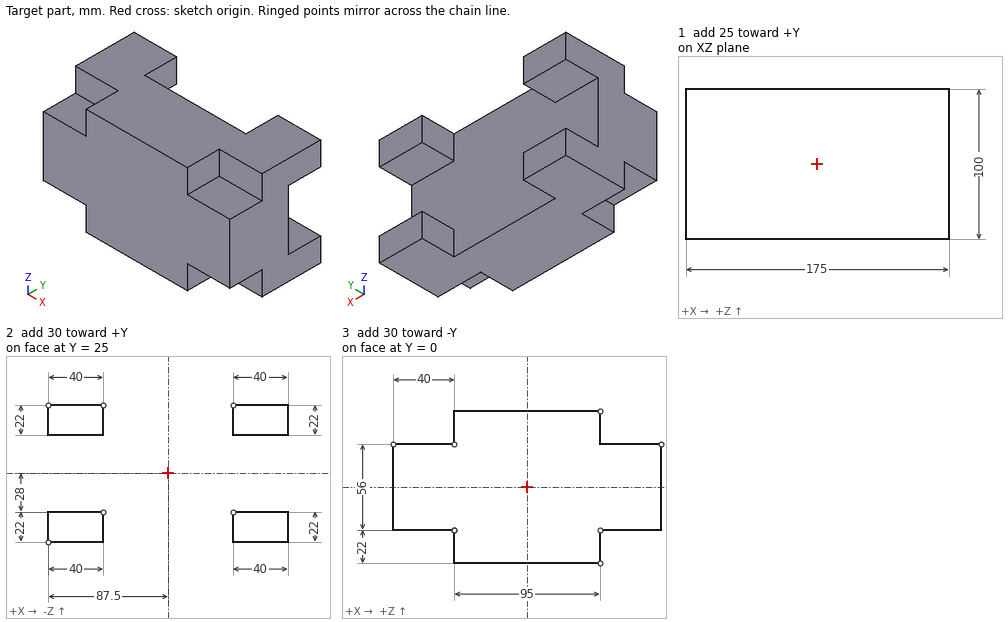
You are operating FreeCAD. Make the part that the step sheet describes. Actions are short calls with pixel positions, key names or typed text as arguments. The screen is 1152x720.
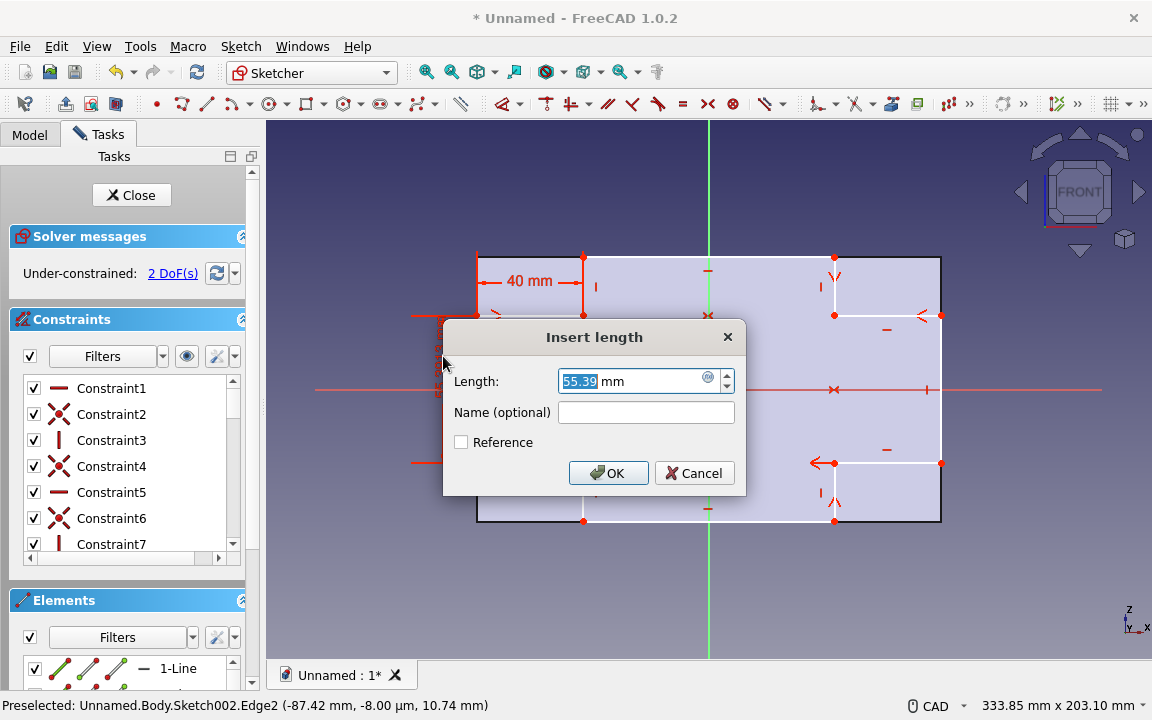
text(56)
key(Return)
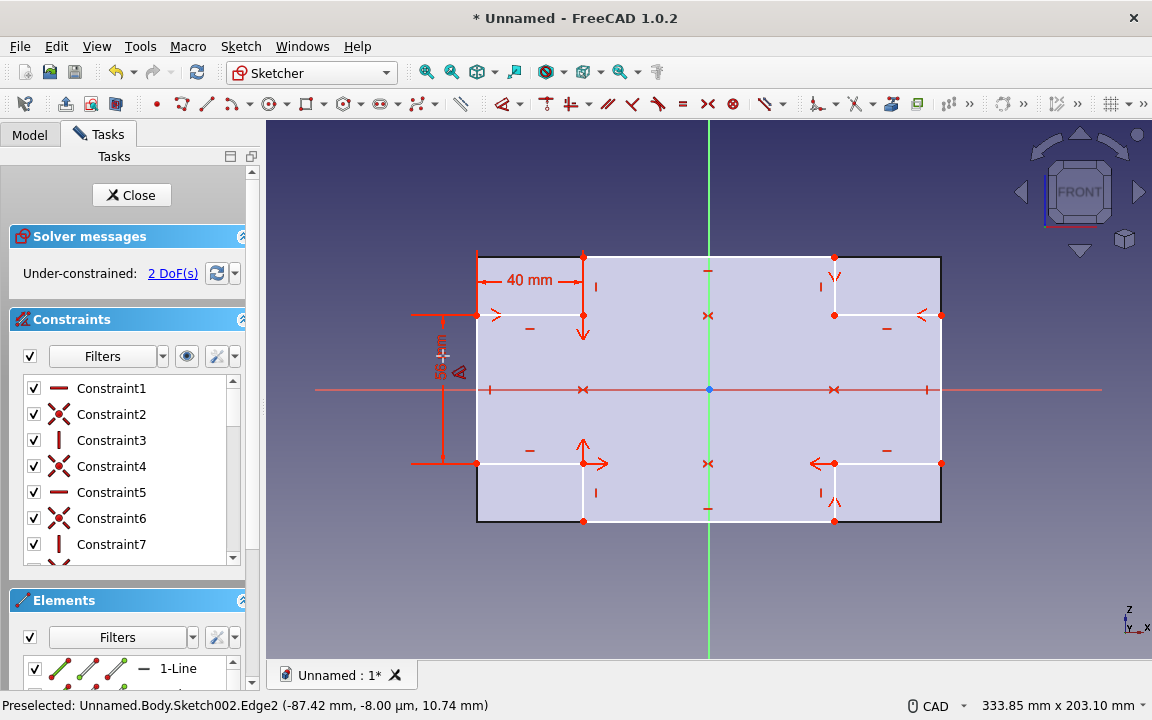
click(583, 481)
click(549, 493)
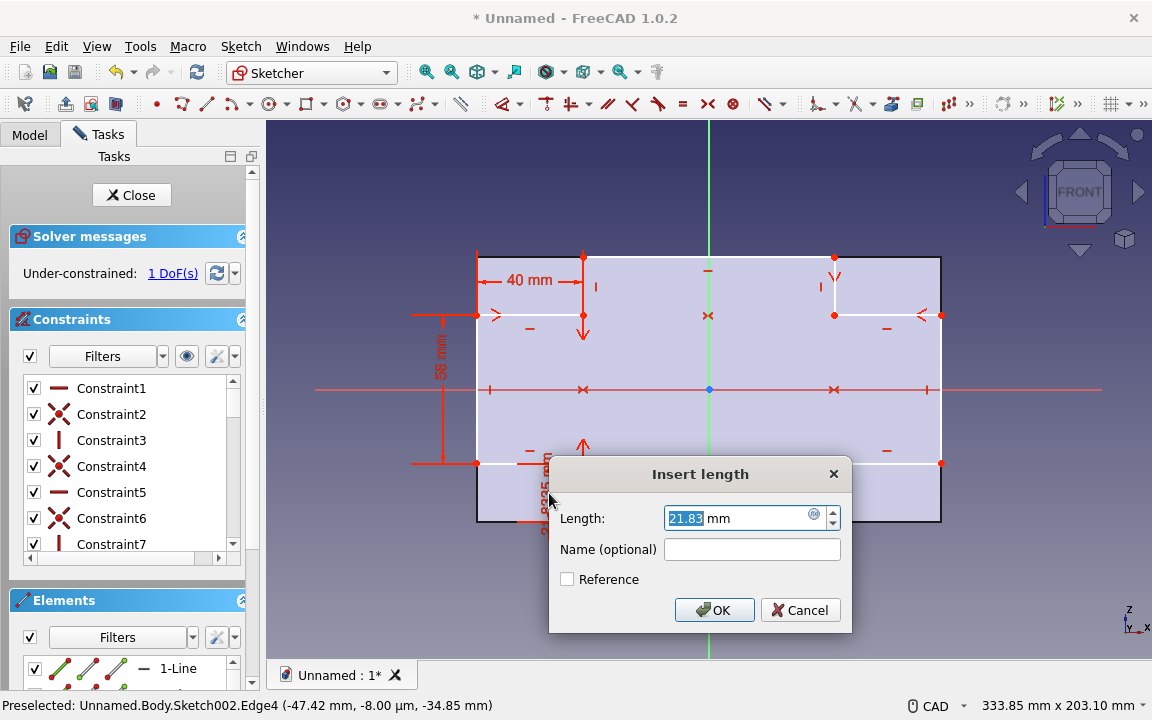
text(22)
key(Return)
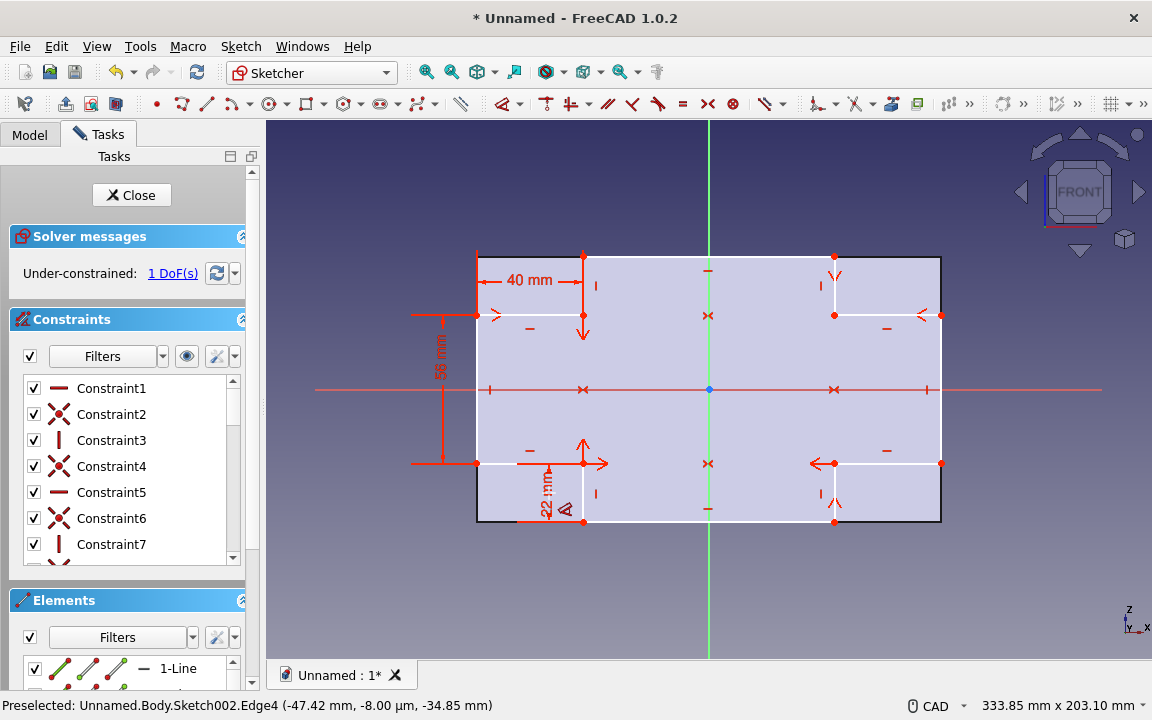
click(659, 522)
click(651, 556)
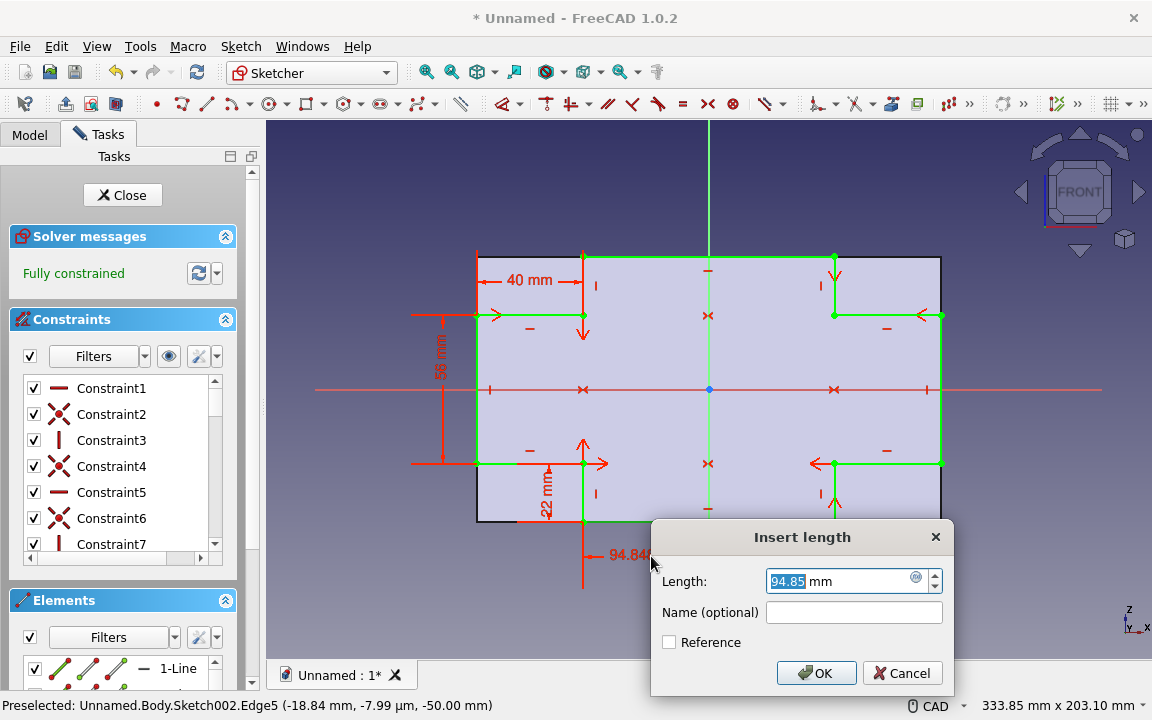
text(95)
key(Return)
key(Escape)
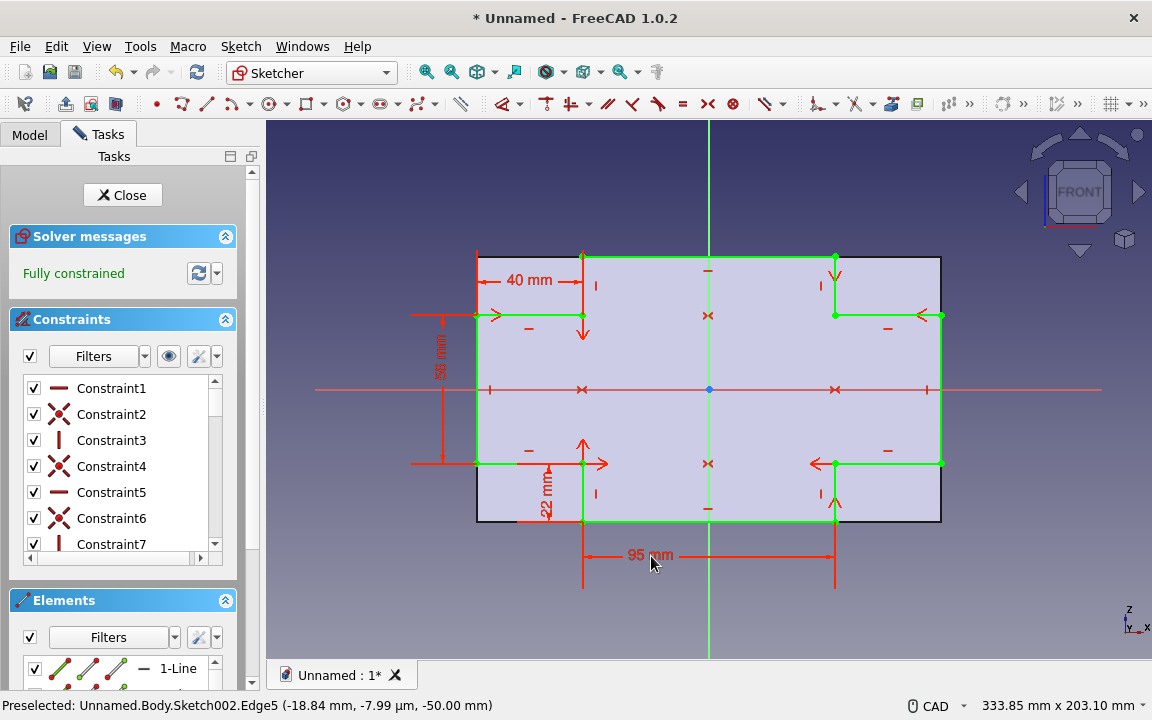
click(123, 195)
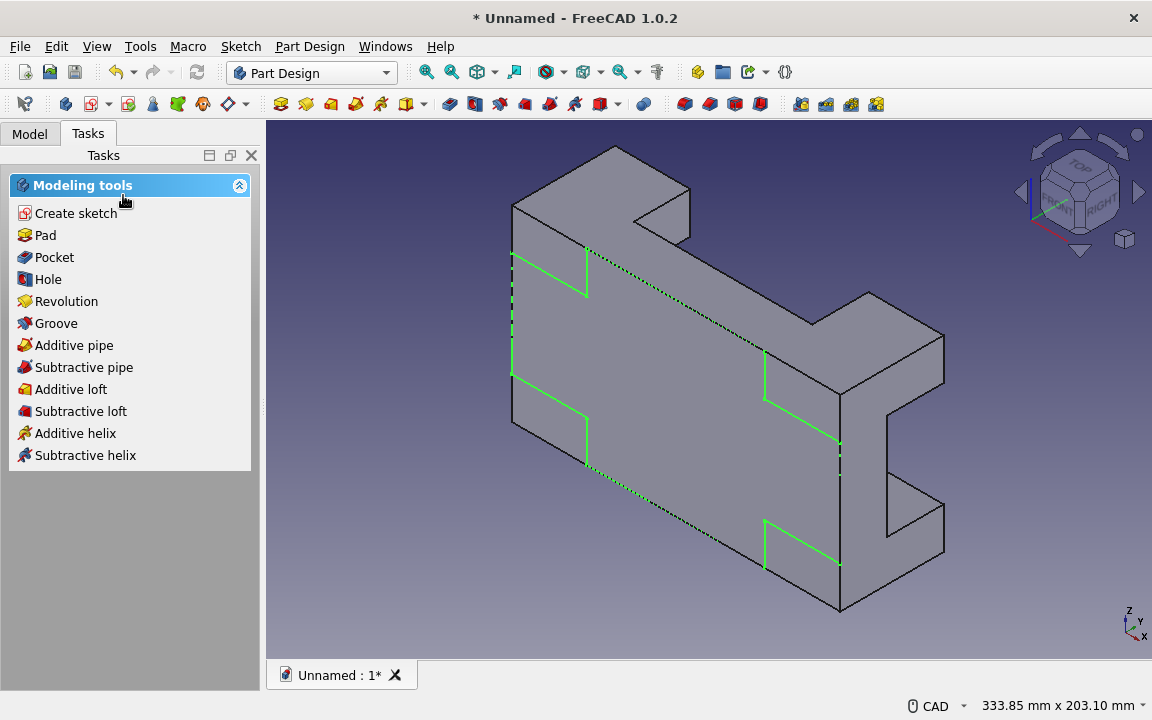
click(281, 104)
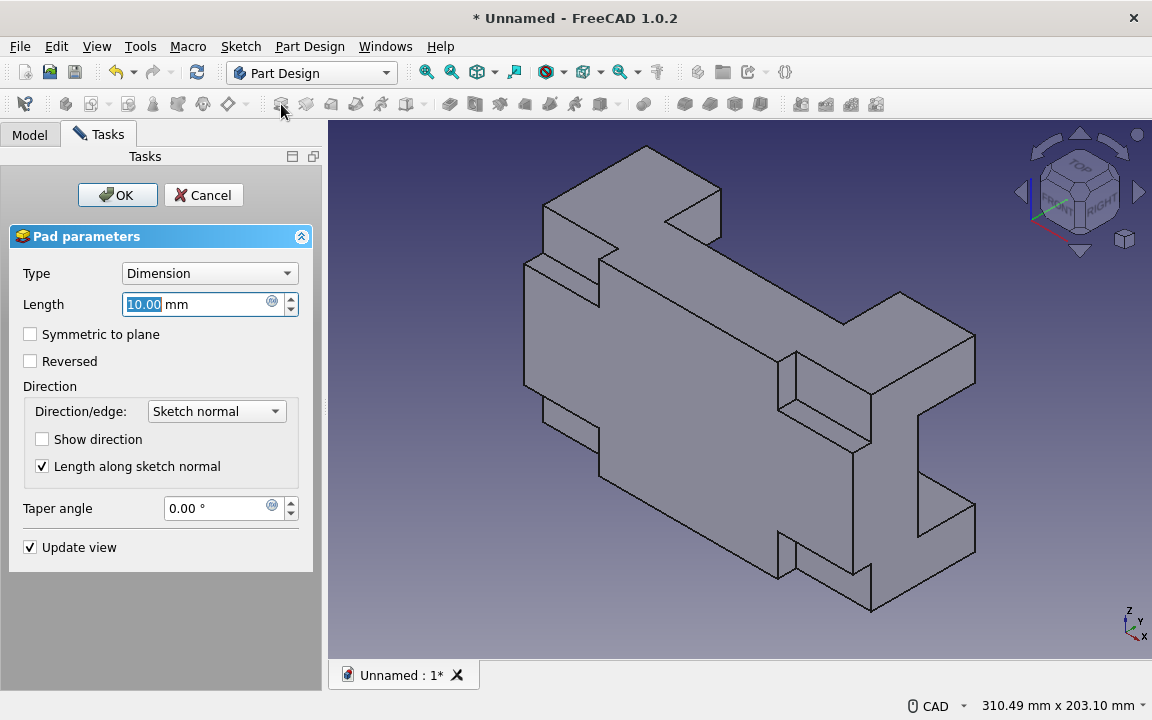
text(30)
key(Tab)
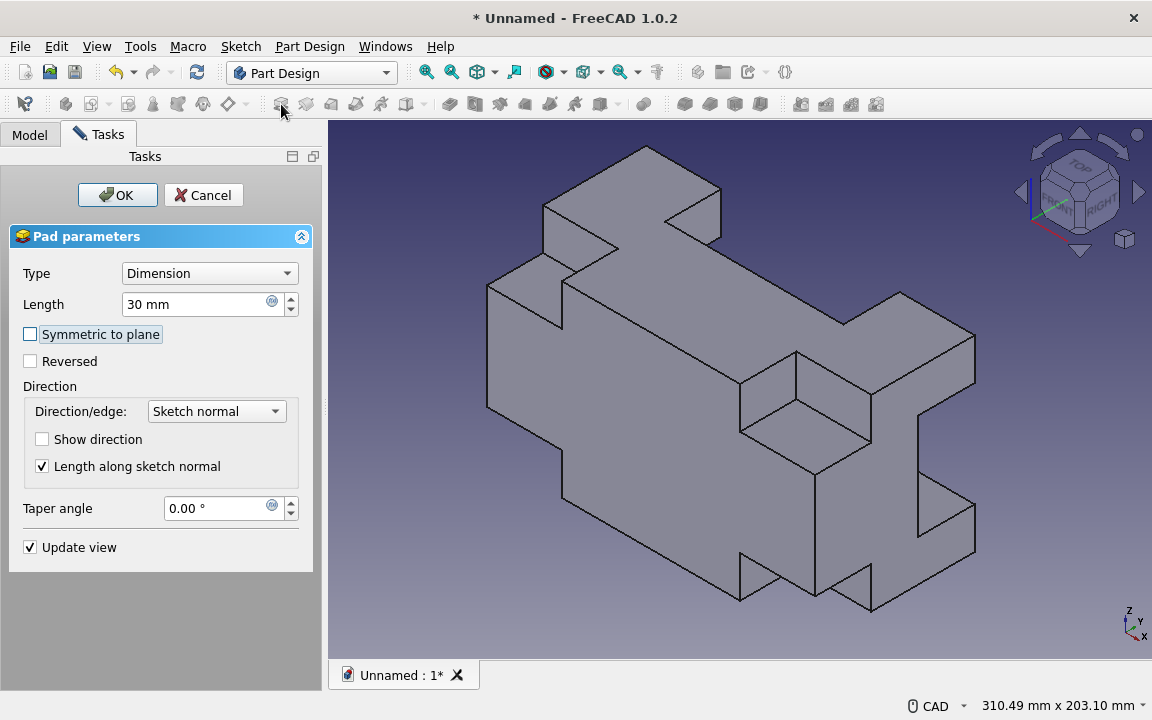
click(118, 195)